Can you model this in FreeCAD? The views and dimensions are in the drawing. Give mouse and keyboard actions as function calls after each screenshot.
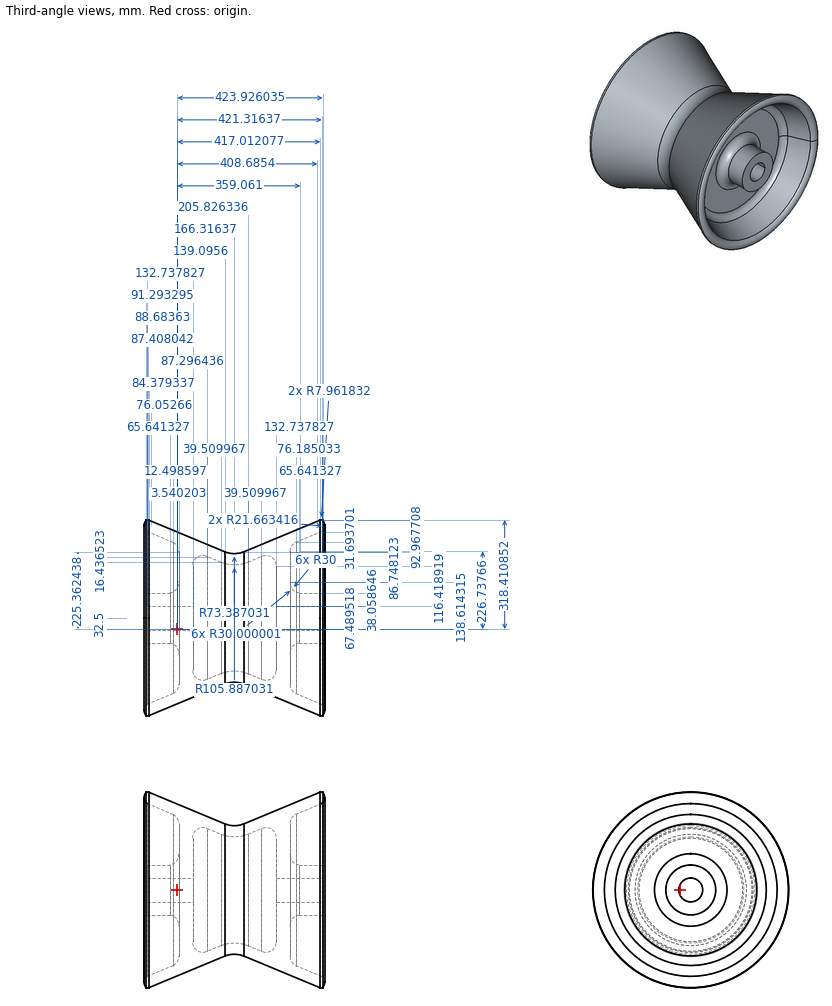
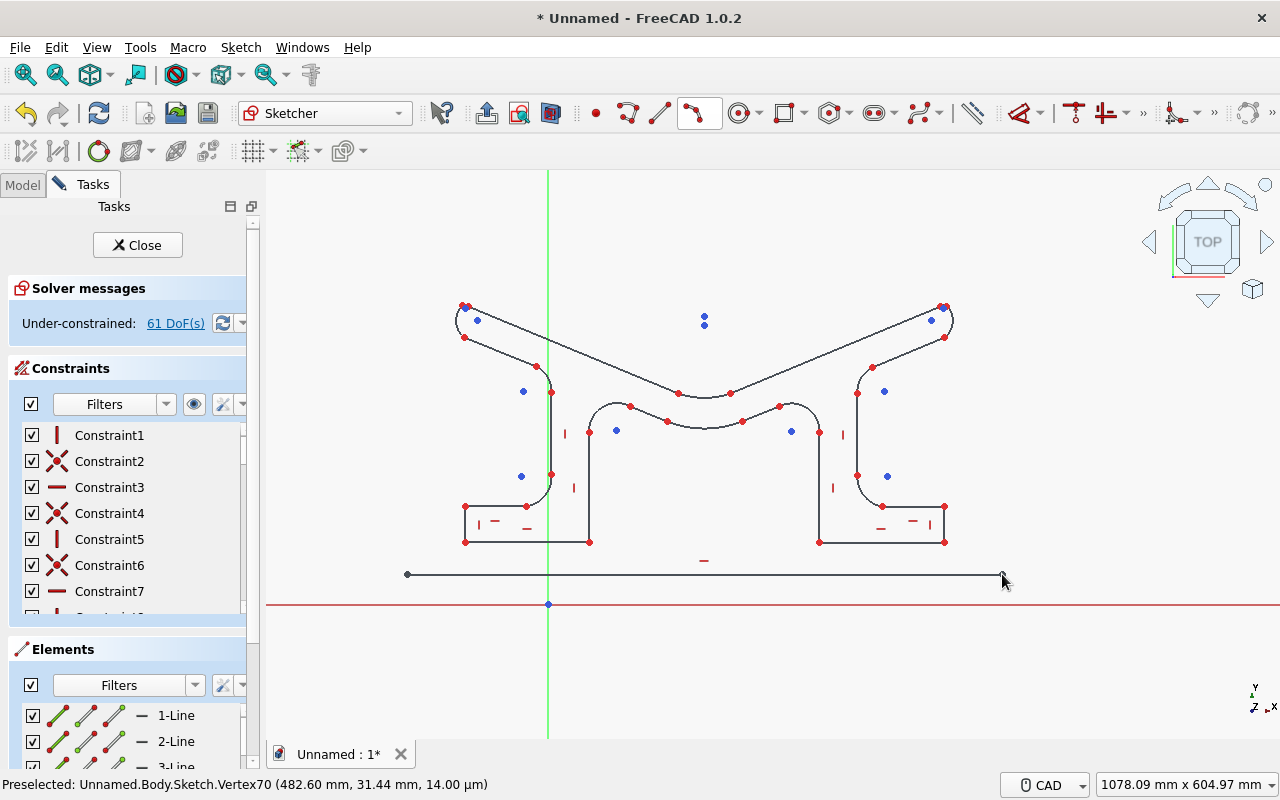
click(585, 575)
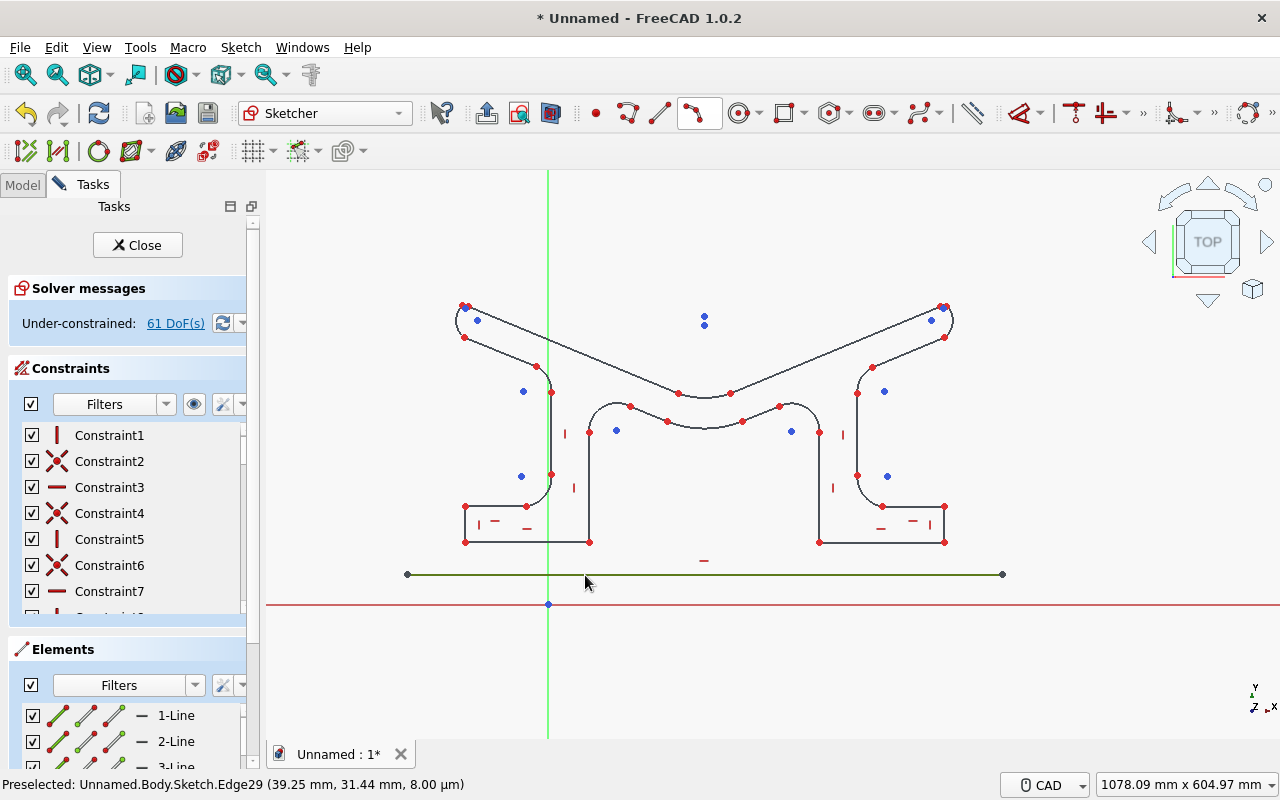
click(974, 114)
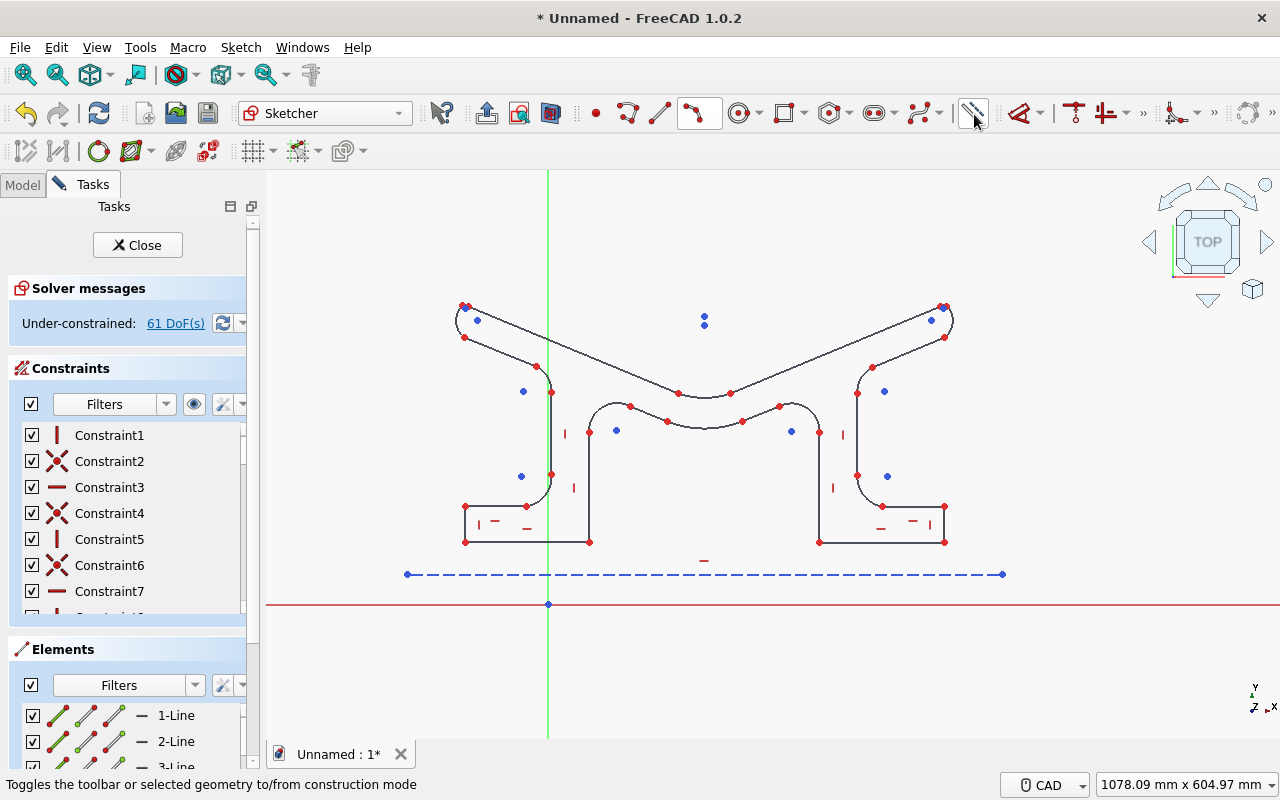
click(694, 397)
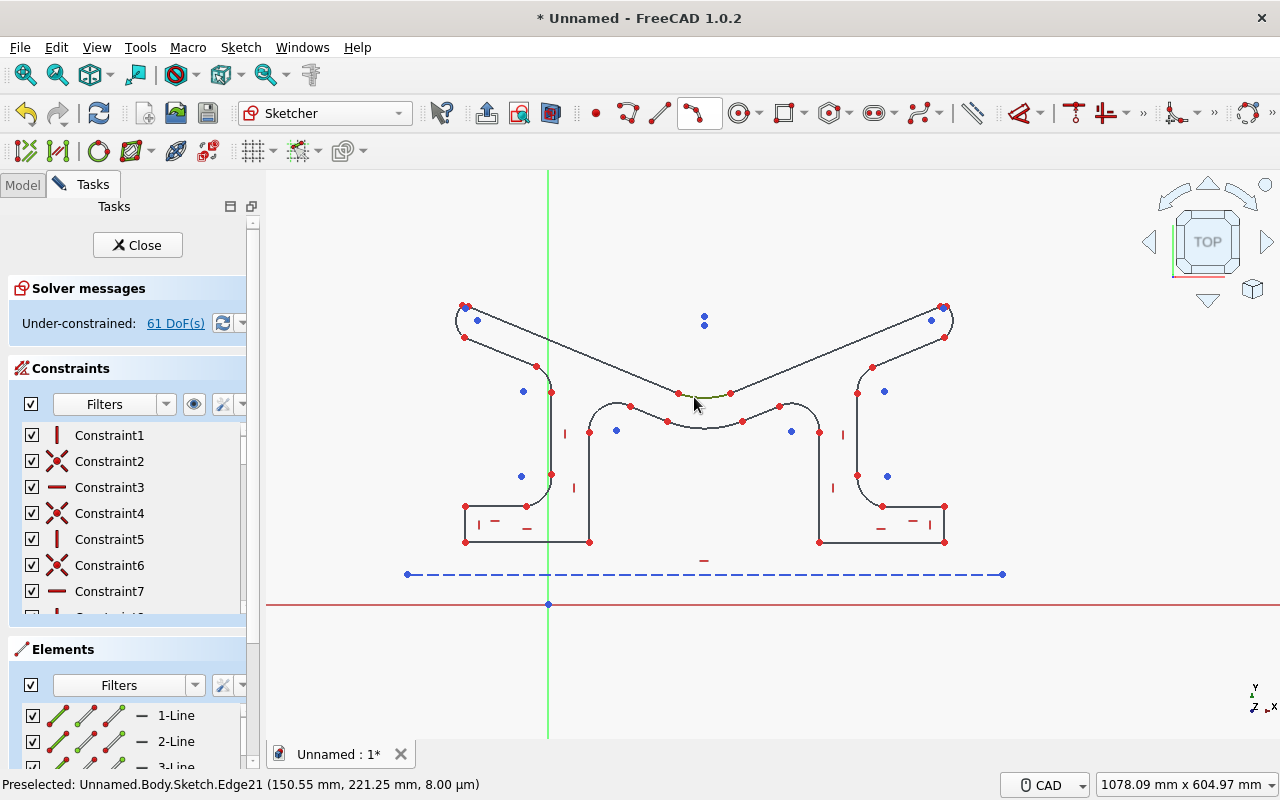
click(689, 427)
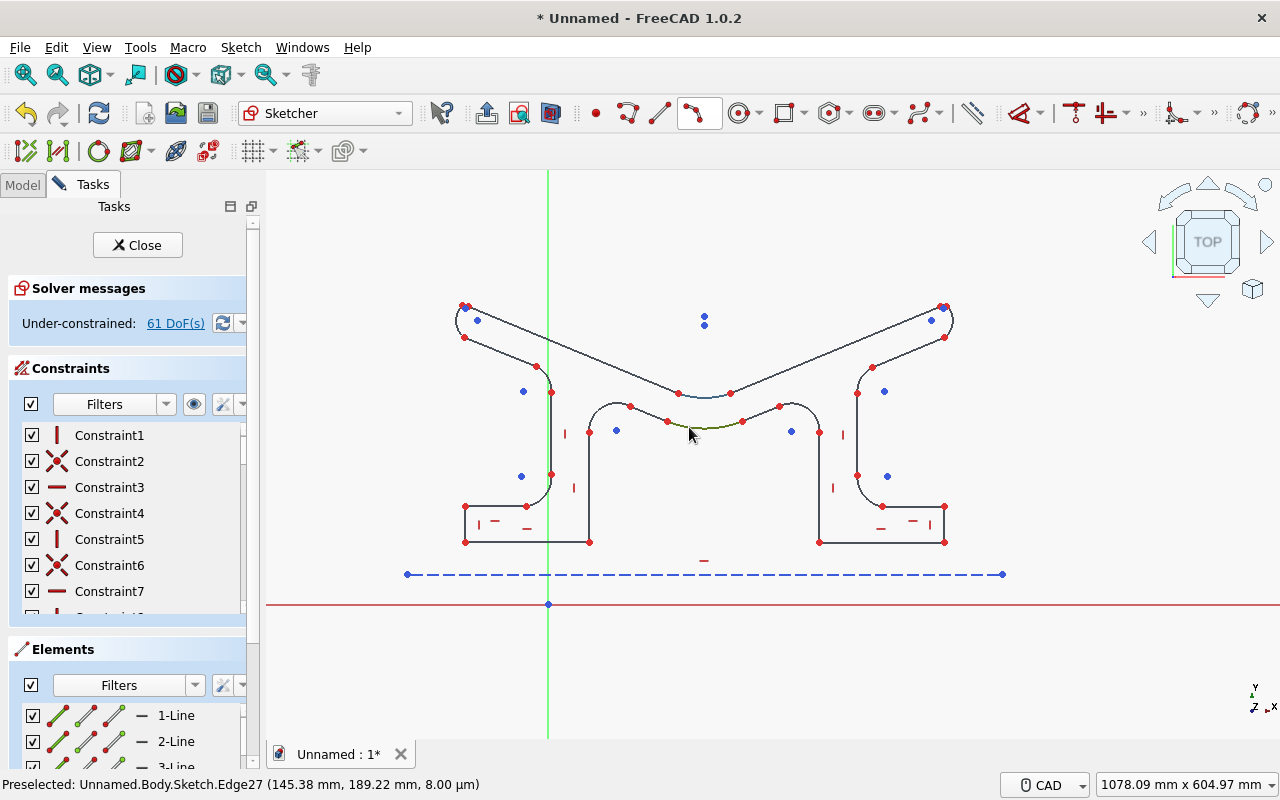
click(1074, 114)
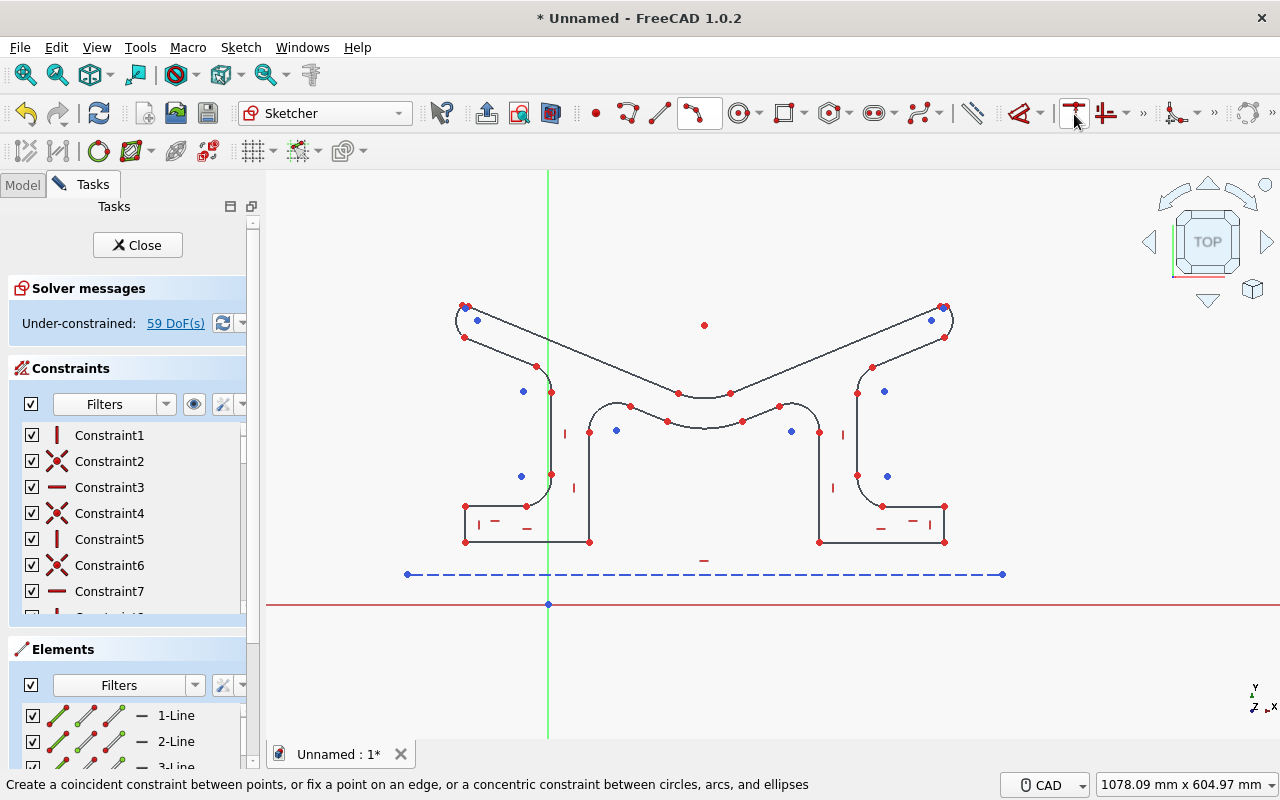
scroll(944, 305, up, 7)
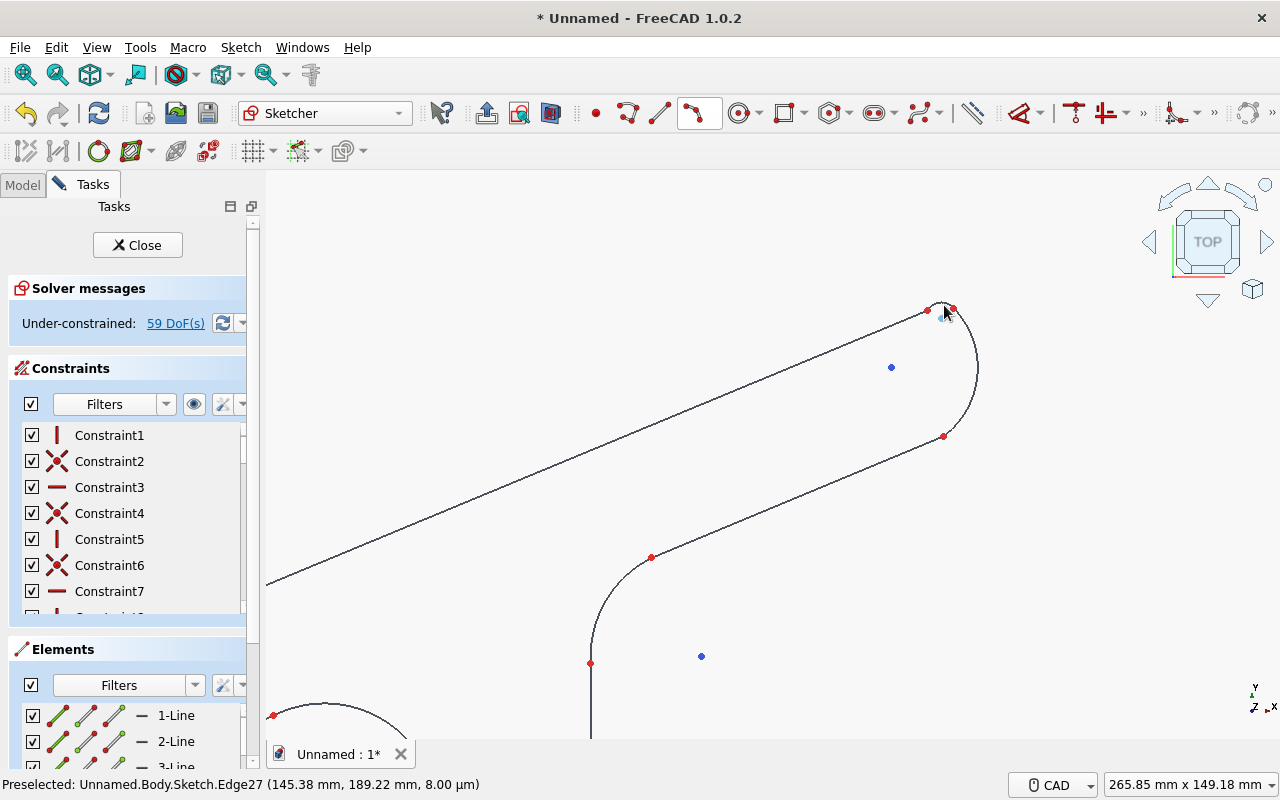
click(940, 303)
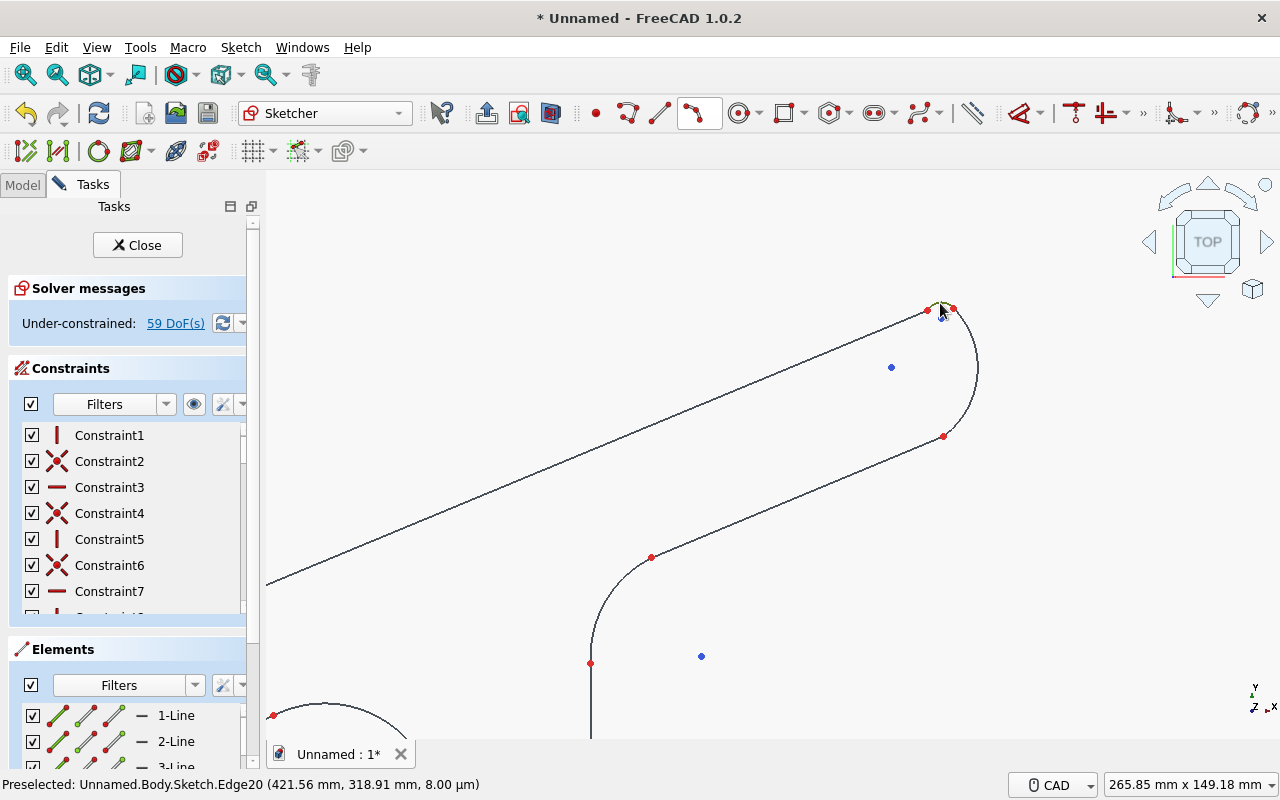
scroll(945, 305, down, 7)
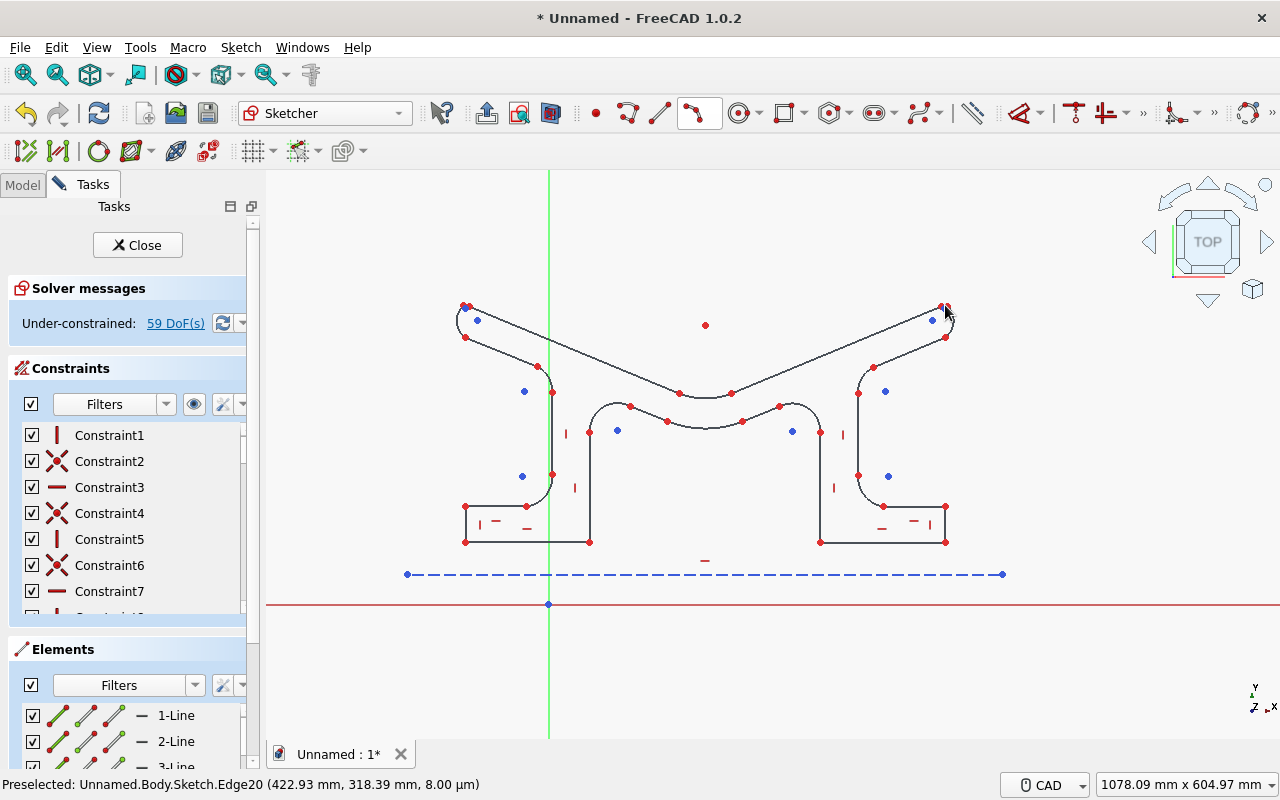
scroll(466, 305, up, 7)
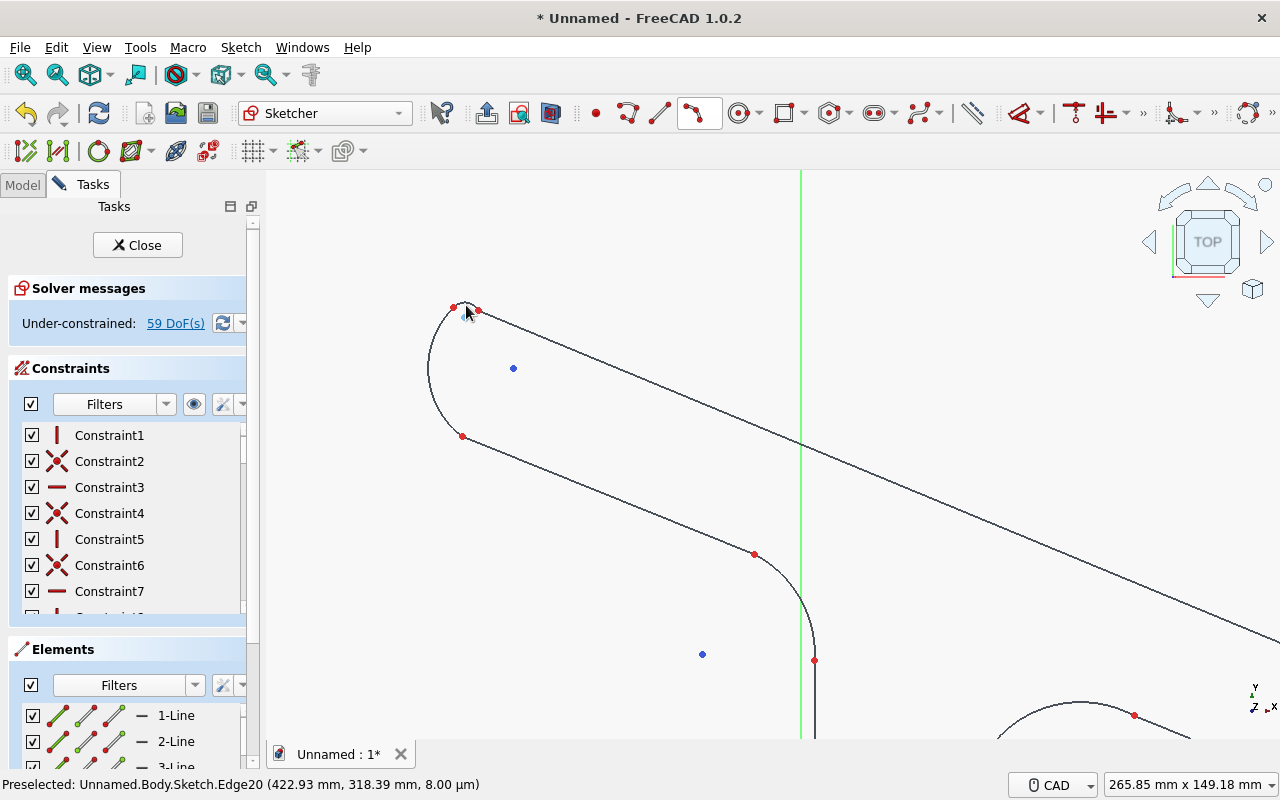
click(467, 303)